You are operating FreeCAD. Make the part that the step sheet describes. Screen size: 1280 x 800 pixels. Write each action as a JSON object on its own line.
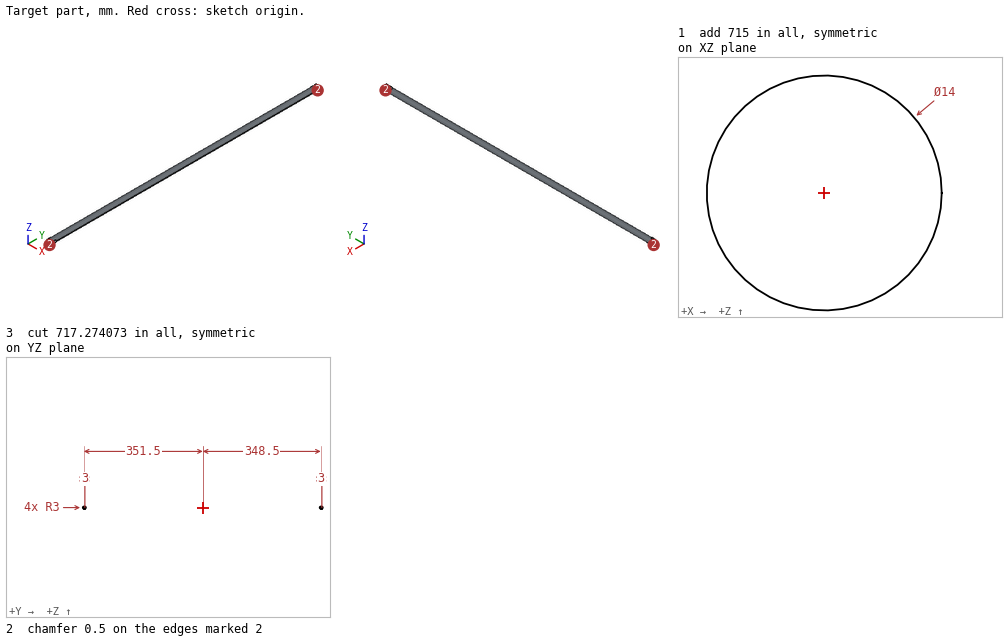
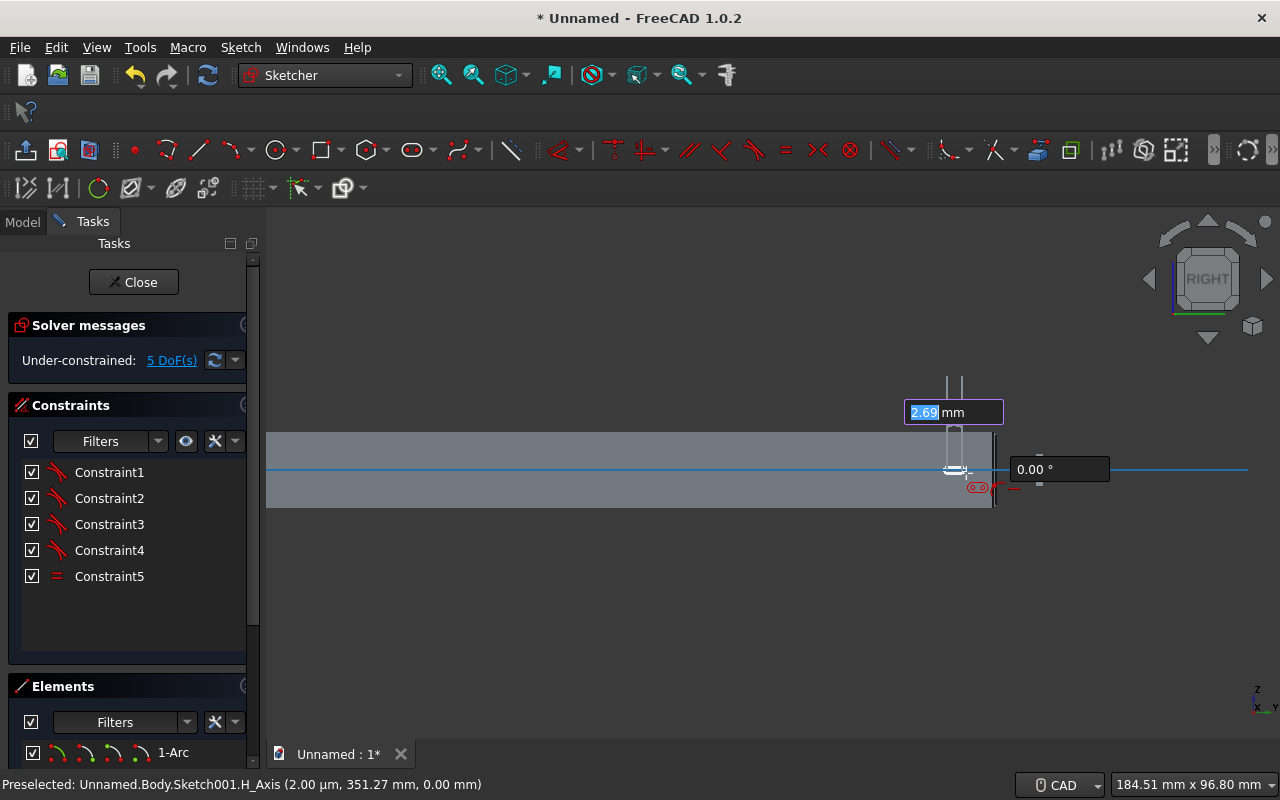
{"action": "left_click", "coordinate": [963, 461]}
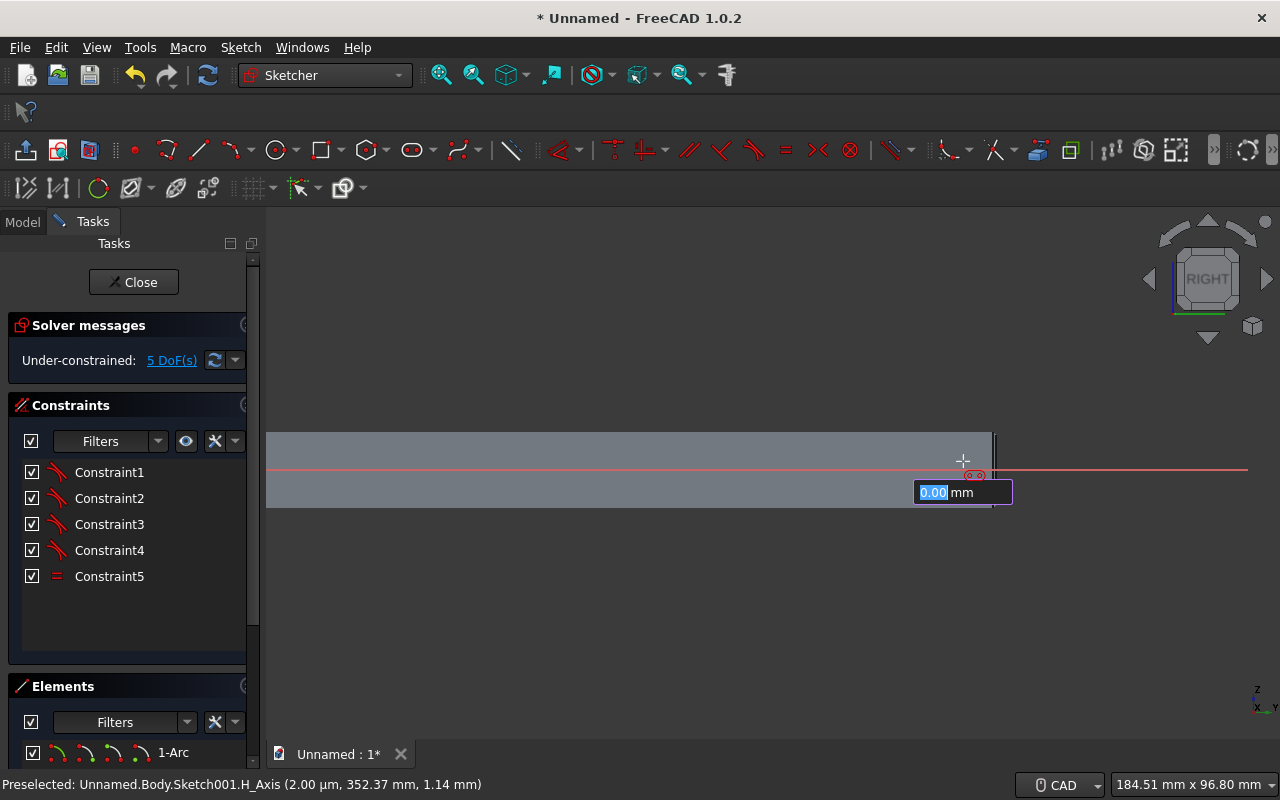
{"action": "left_click", "coordinate": [955, 454]}
{"action": "key", "text": "Escape"}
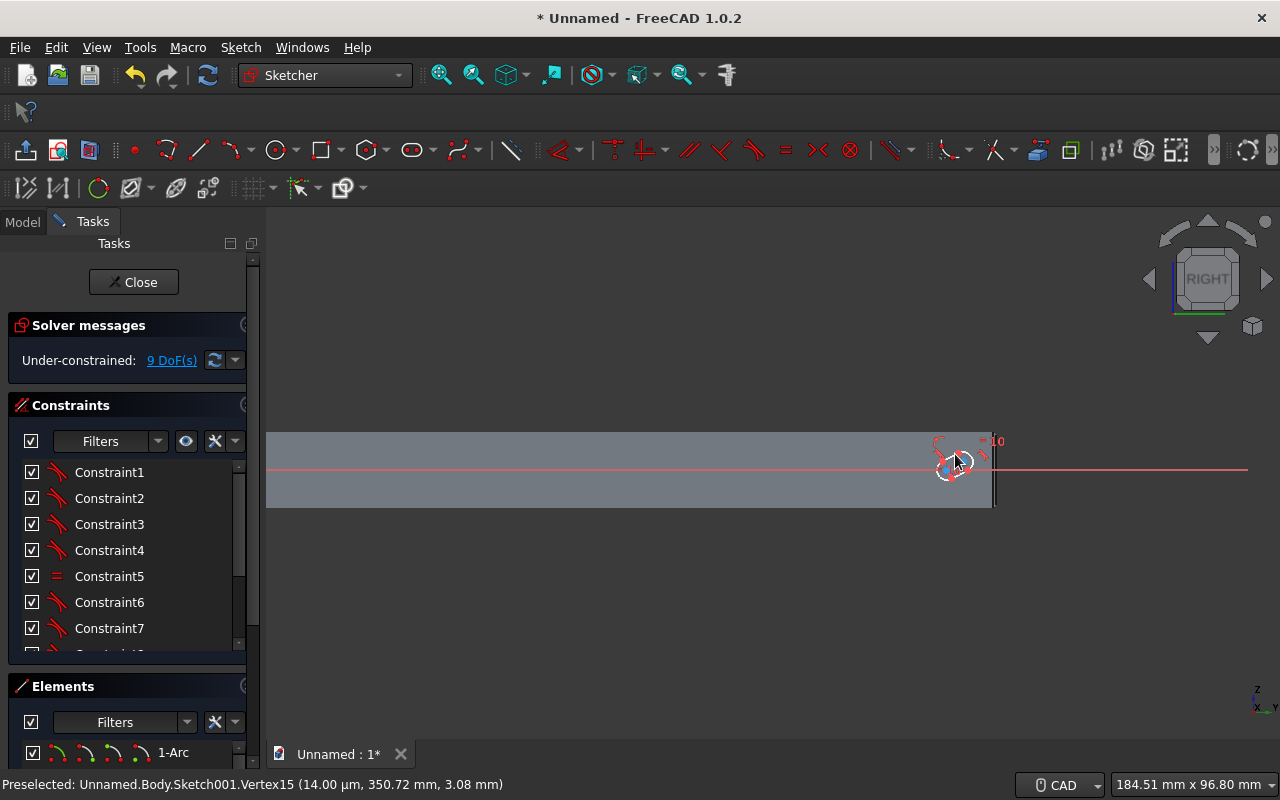
{"action": "scroll", "coordinate": [966, 473], "scroll_direction": "down", "scroll_amount": 10}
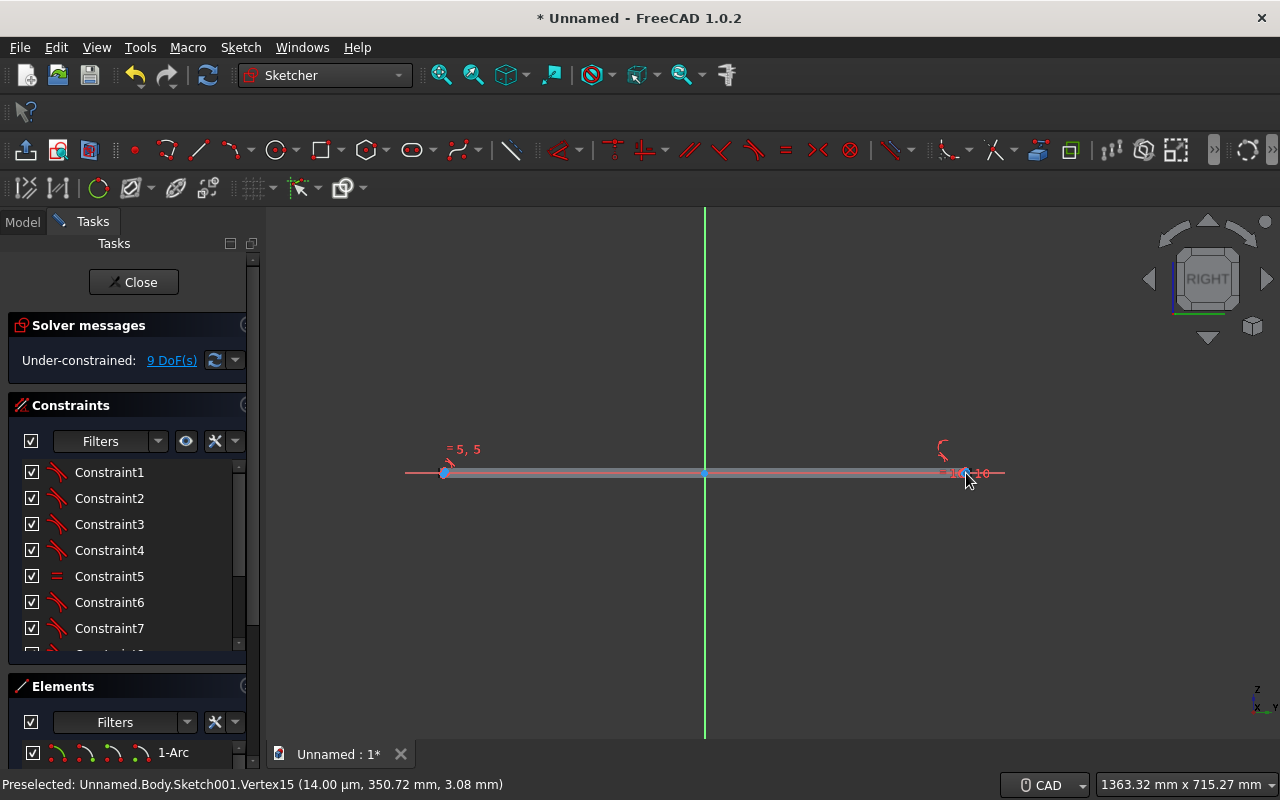
{"action": "scroll", "coordinate": [444, 472], "scroll_direction": "up", "scroll_amount": 12}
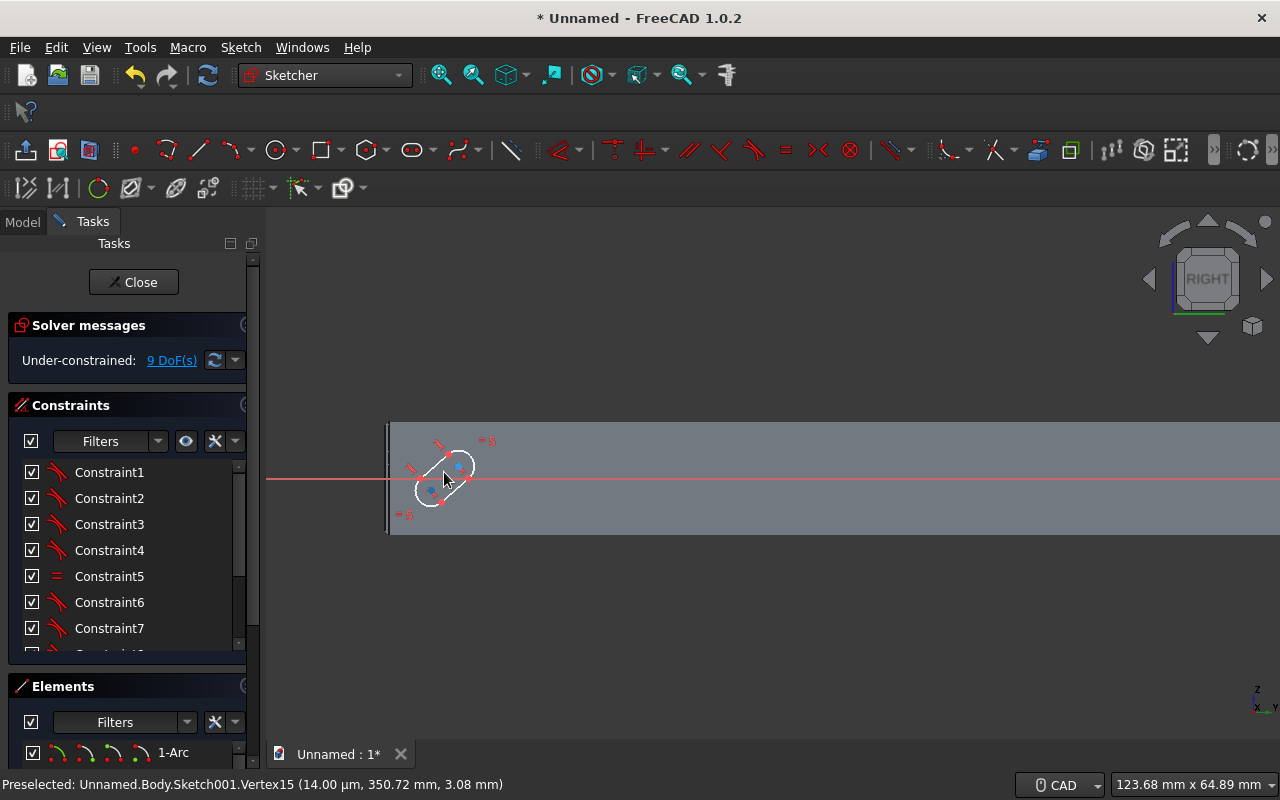
{"action": "left_click", "coordinate": [437, 464]}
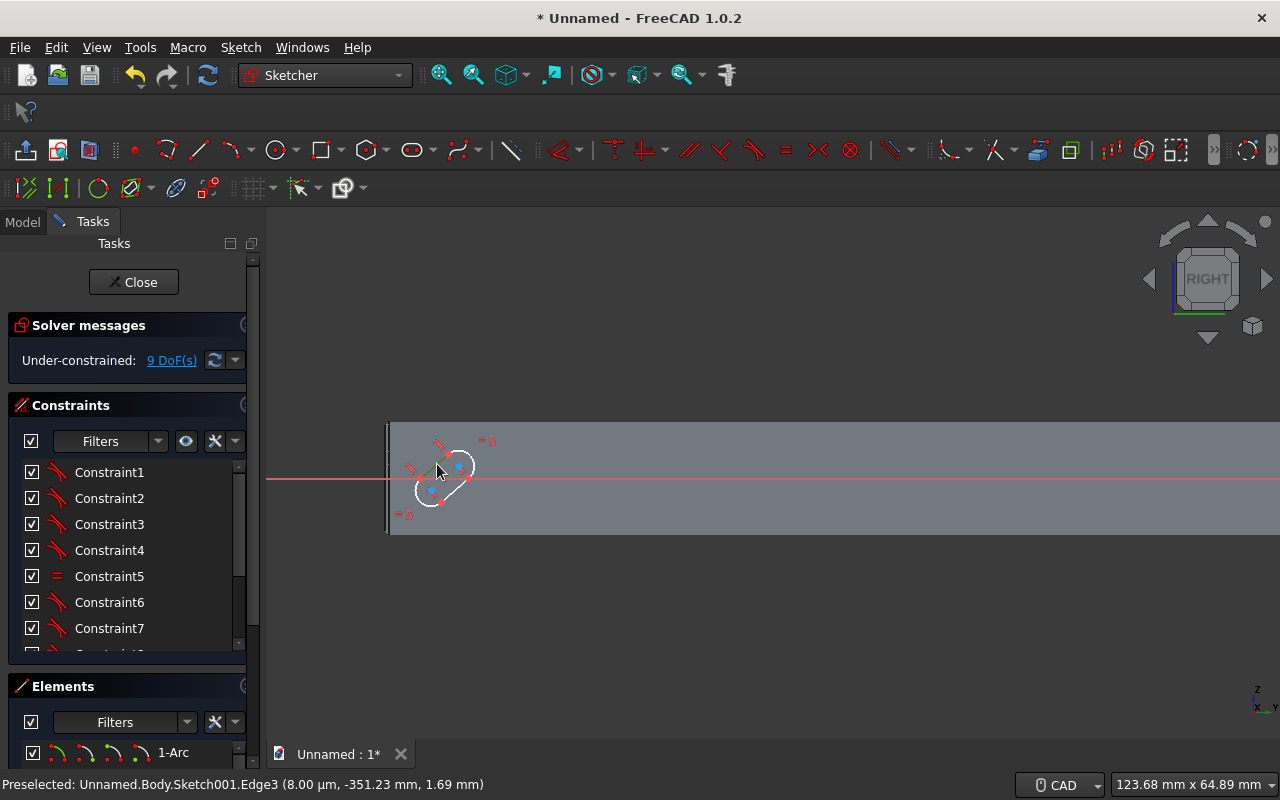
{"action": "key", "text": "h"}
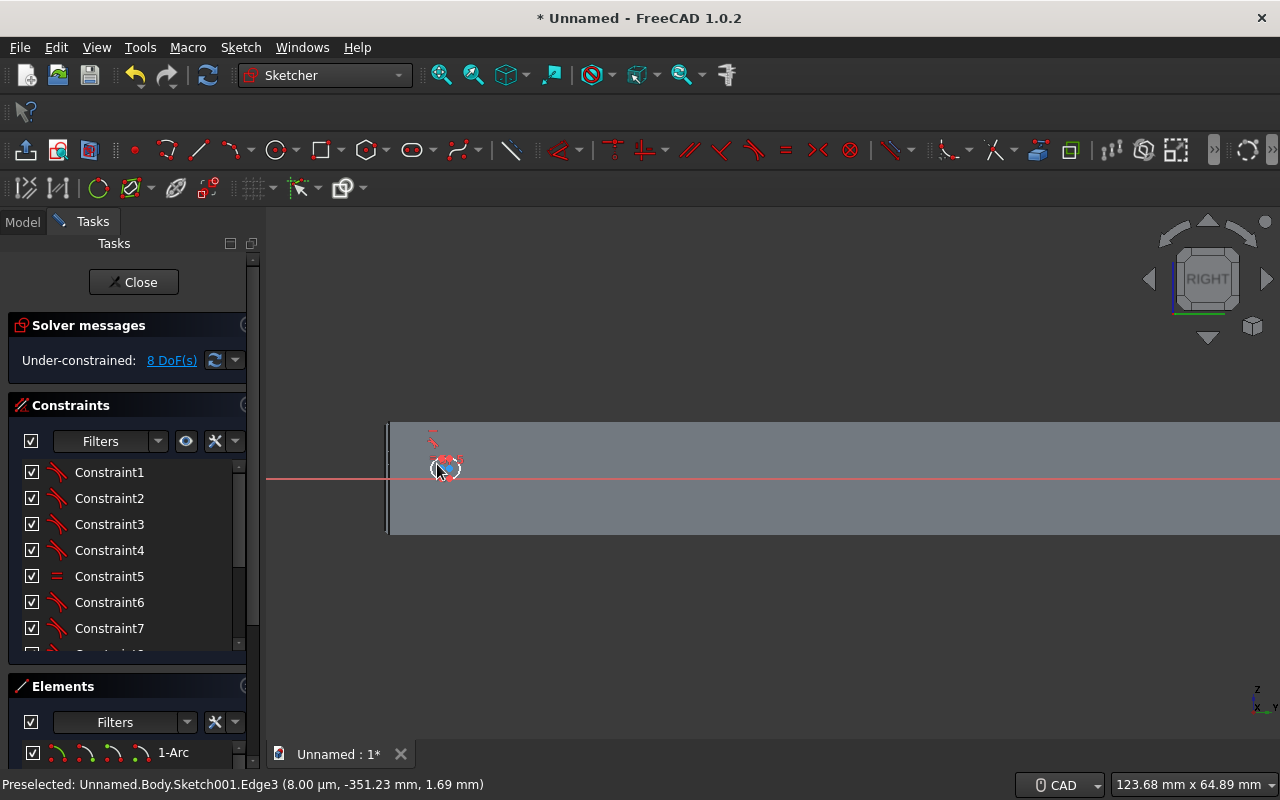
{"action": "scroll", "coordinate": [444, 472], "scroll_direction": "down", "scroll_amount": 12}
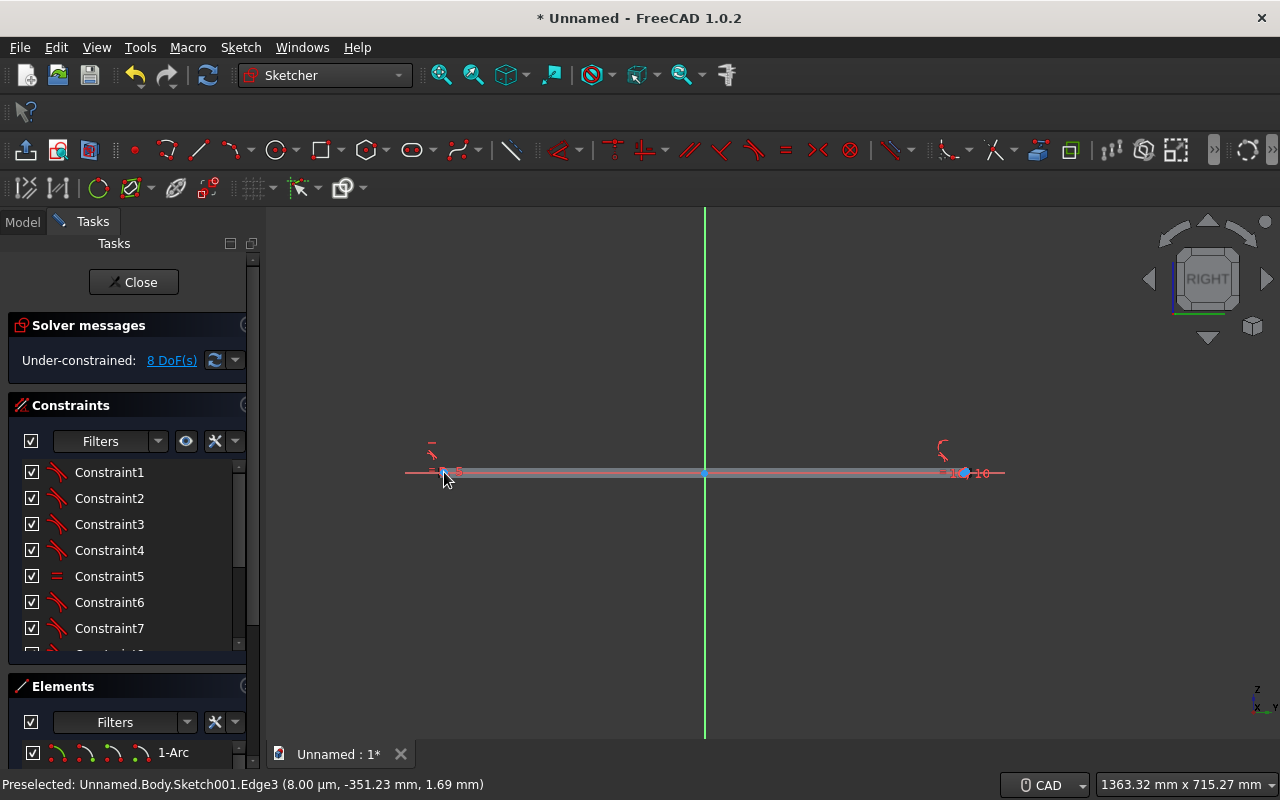
{"action": "scroll", "coordinate": [964, 471], "scroll_direction": "up", "scroll_amount": 14}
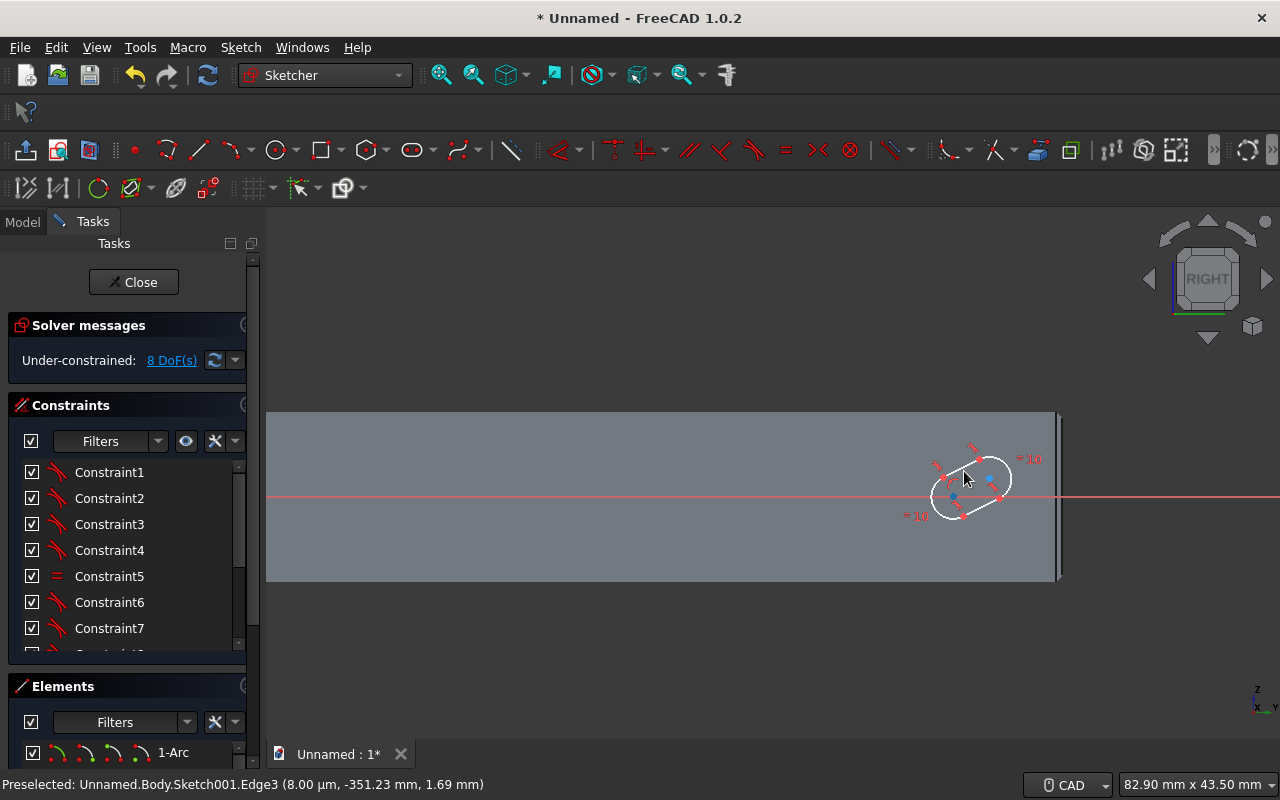
{"action": "left_click", "coordinate": [958, 470]}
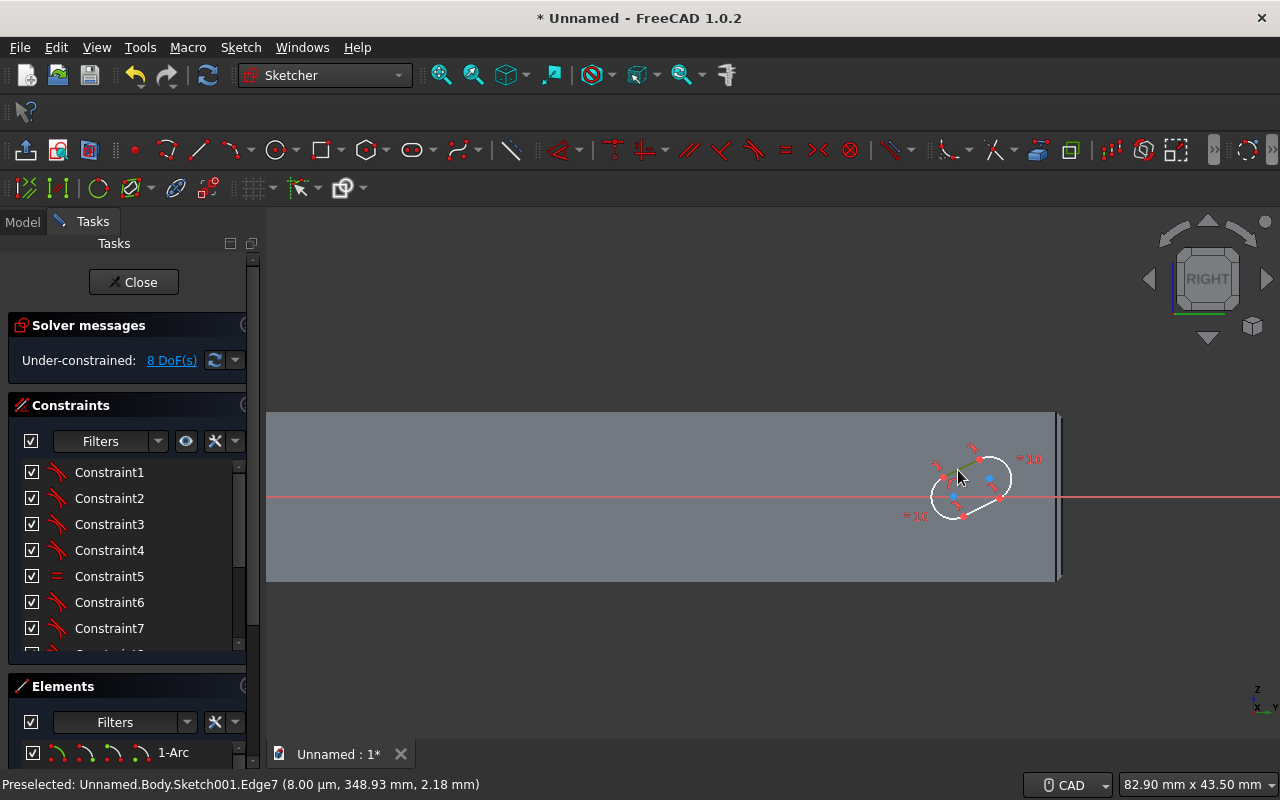
{"action": "key", "text": "h"}